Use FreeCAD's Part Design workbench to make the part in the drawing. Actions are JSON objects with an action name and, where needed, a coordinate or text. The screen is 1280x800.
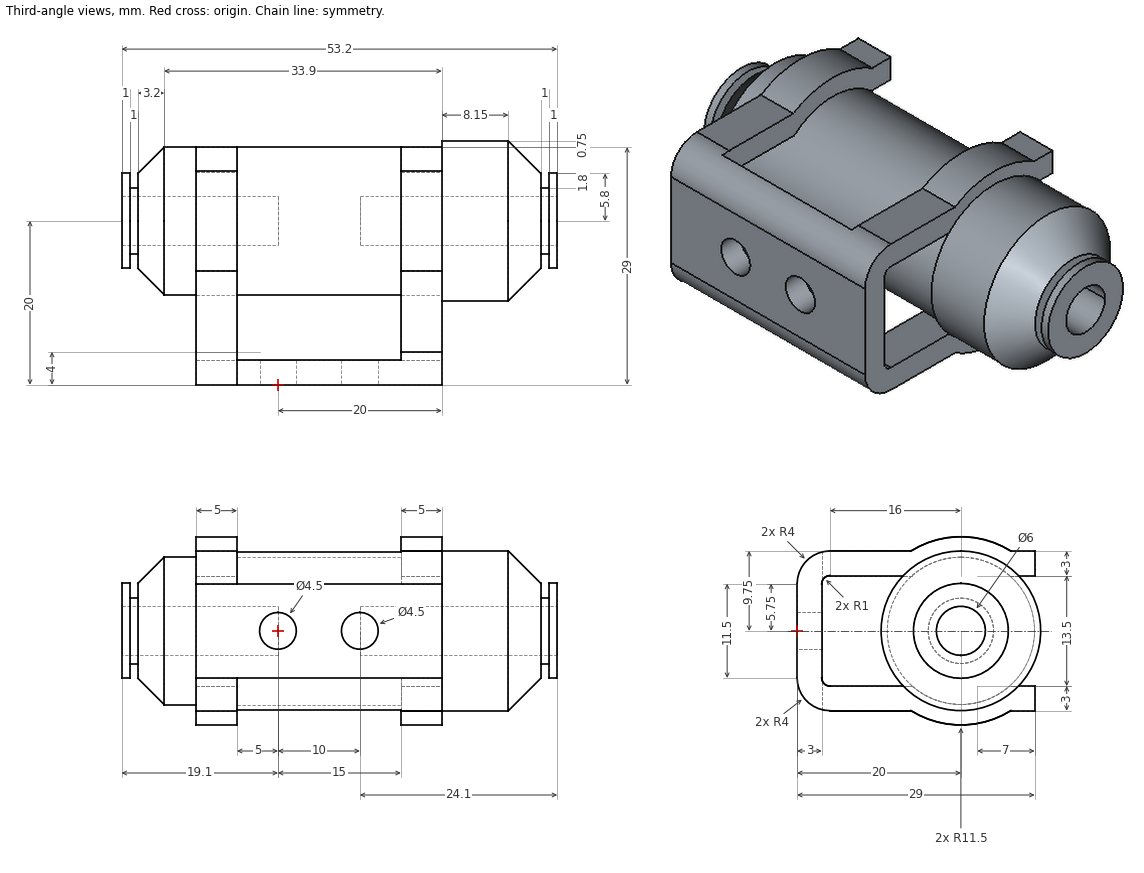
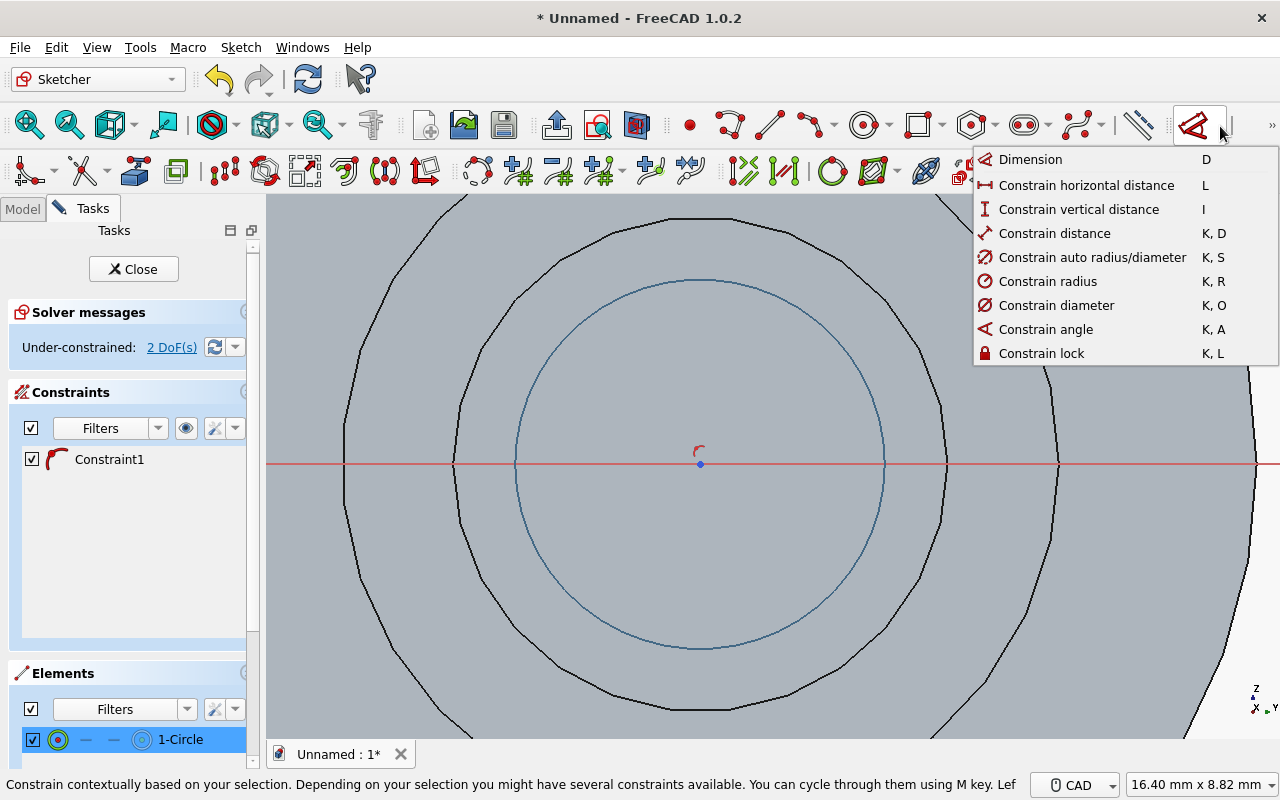
{"action": "left_click", "coordinate": [1126, 305]}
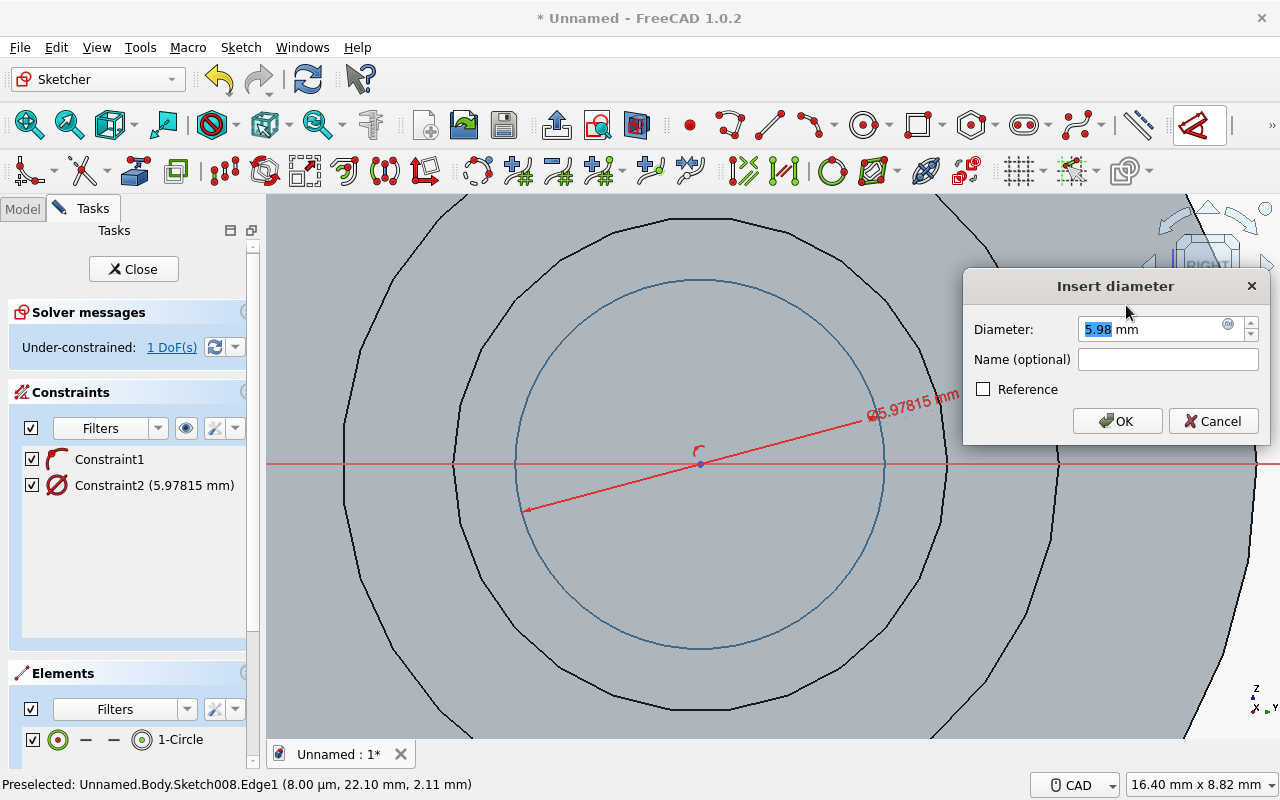
{"action": "type", "text": "6"}
{"action": "key", "text": "Return"}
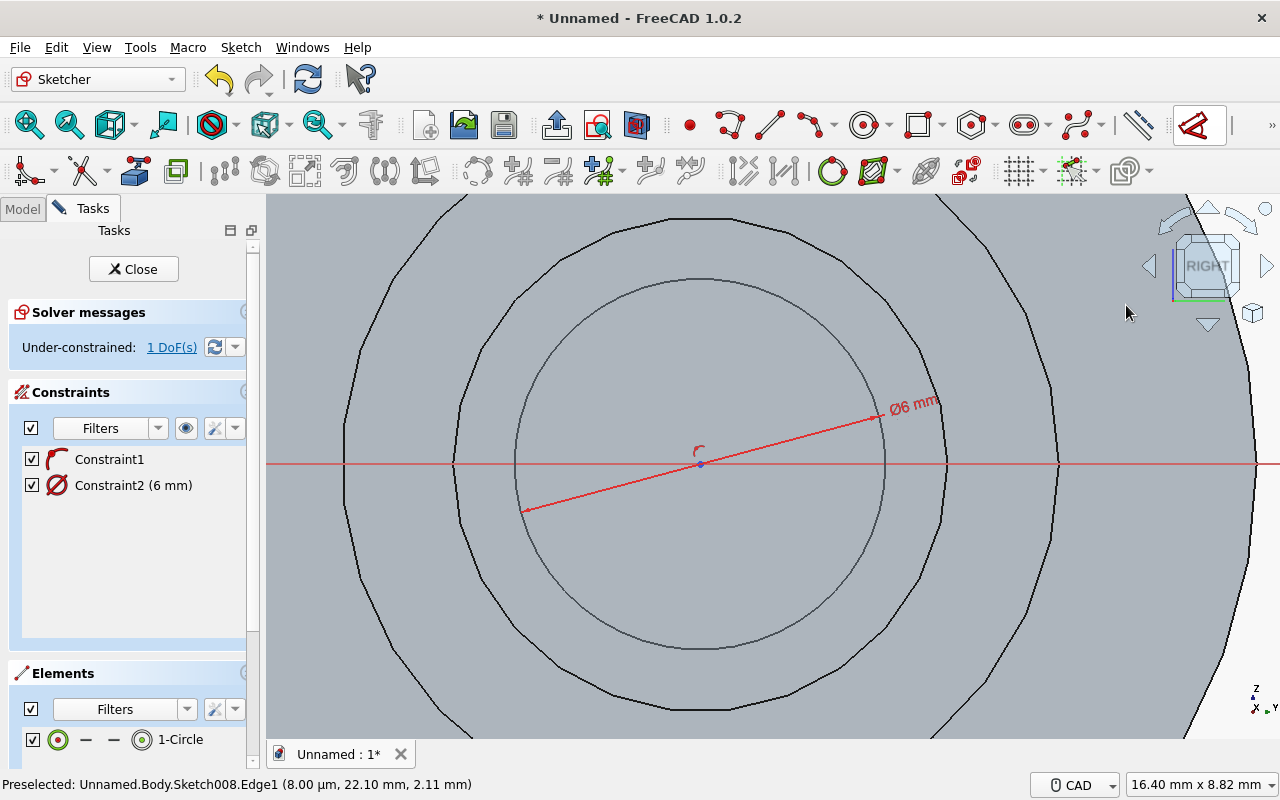
{"action": "left_click", "coordinate": [700, 464]}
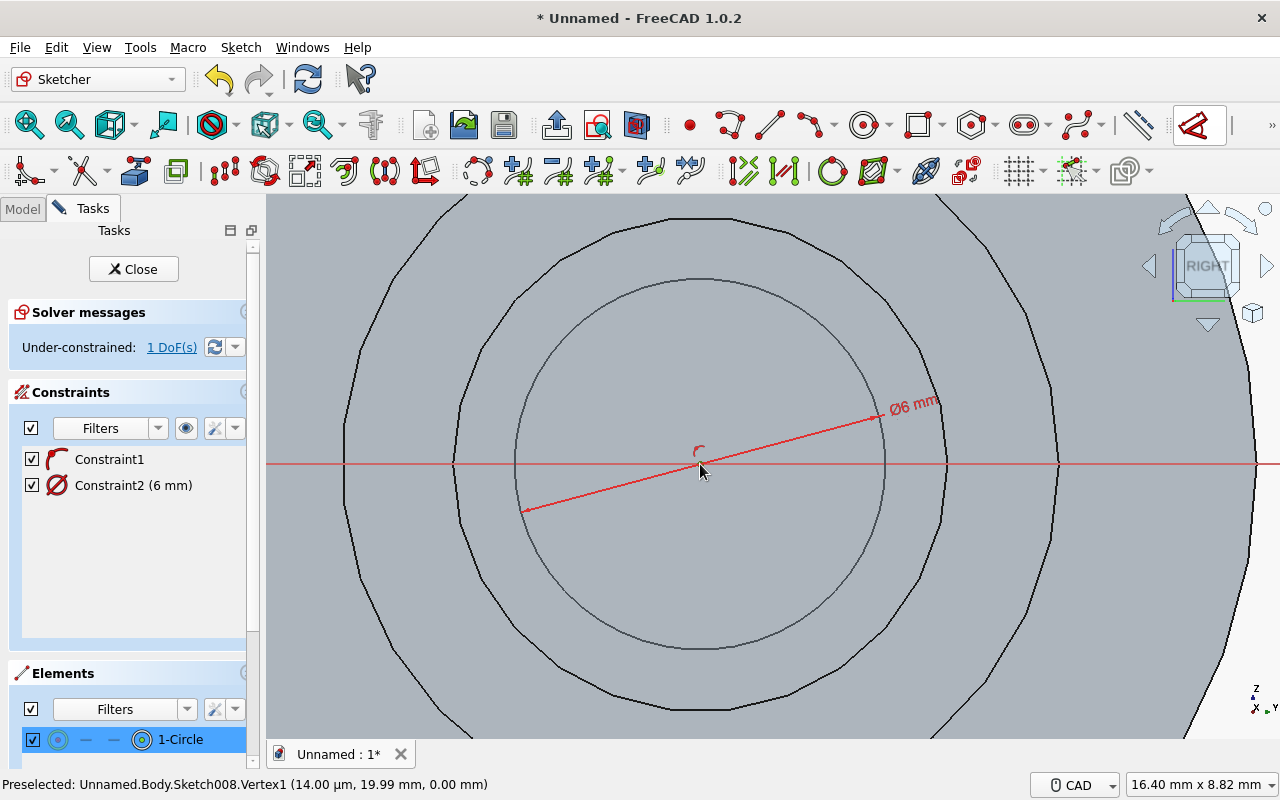
{"action": "left_click", "coordinate": [1220, 126]}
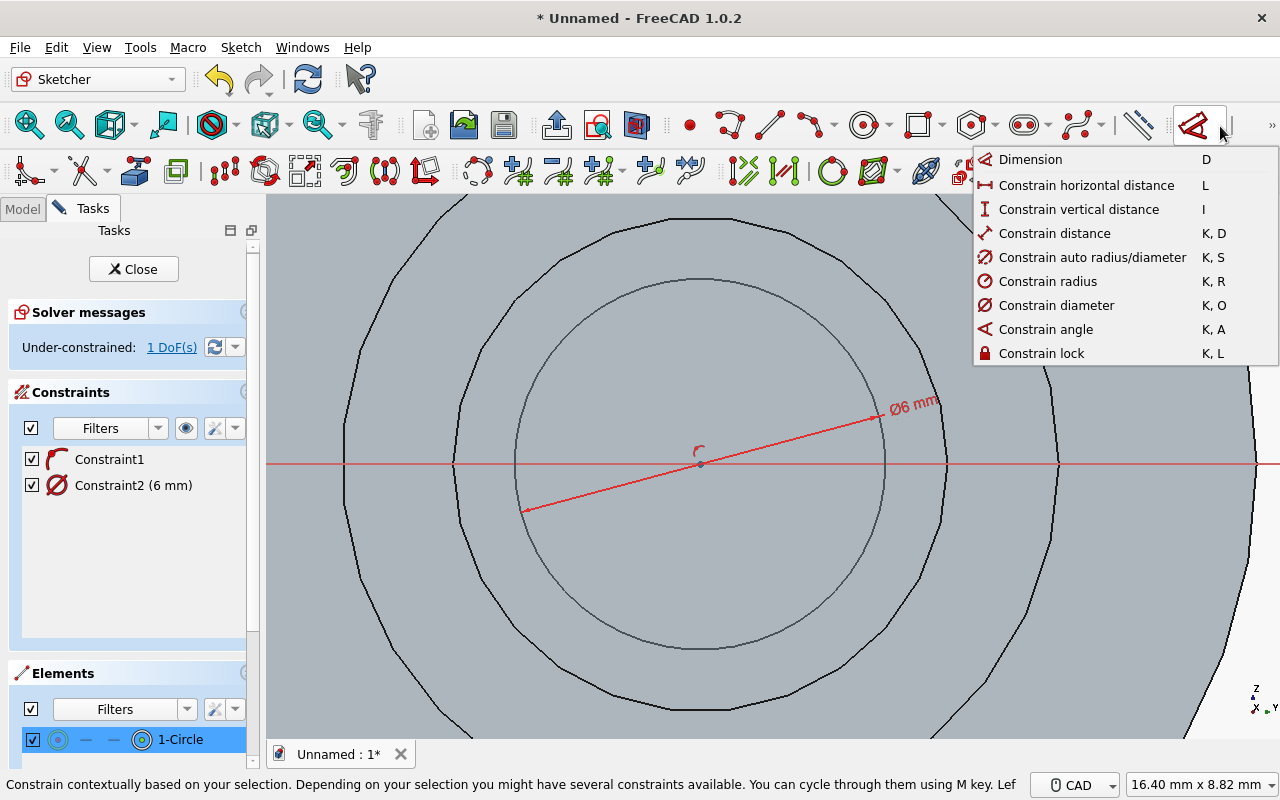
{"action": "left_click", "coordinate": [1126, 185]}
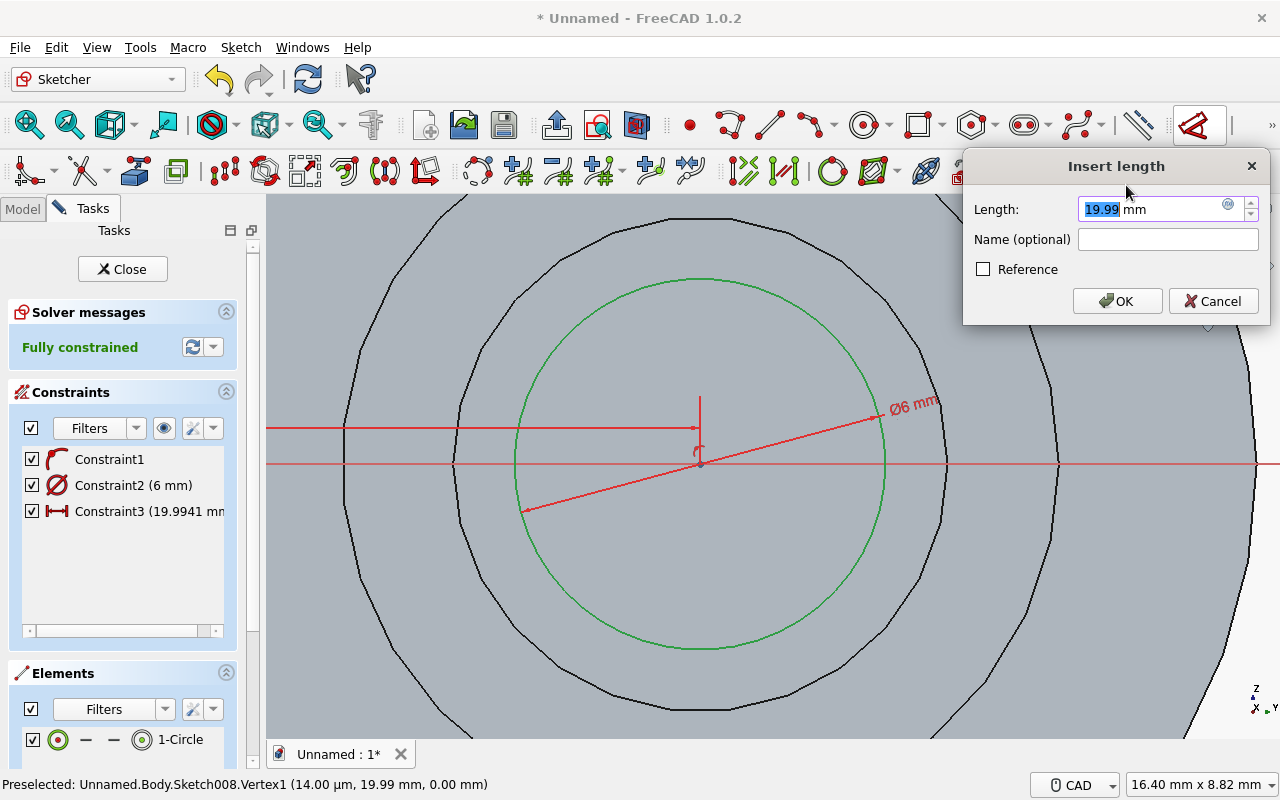
{"action": "type", "text": "20"}
{"action": "key", "text": "Return"}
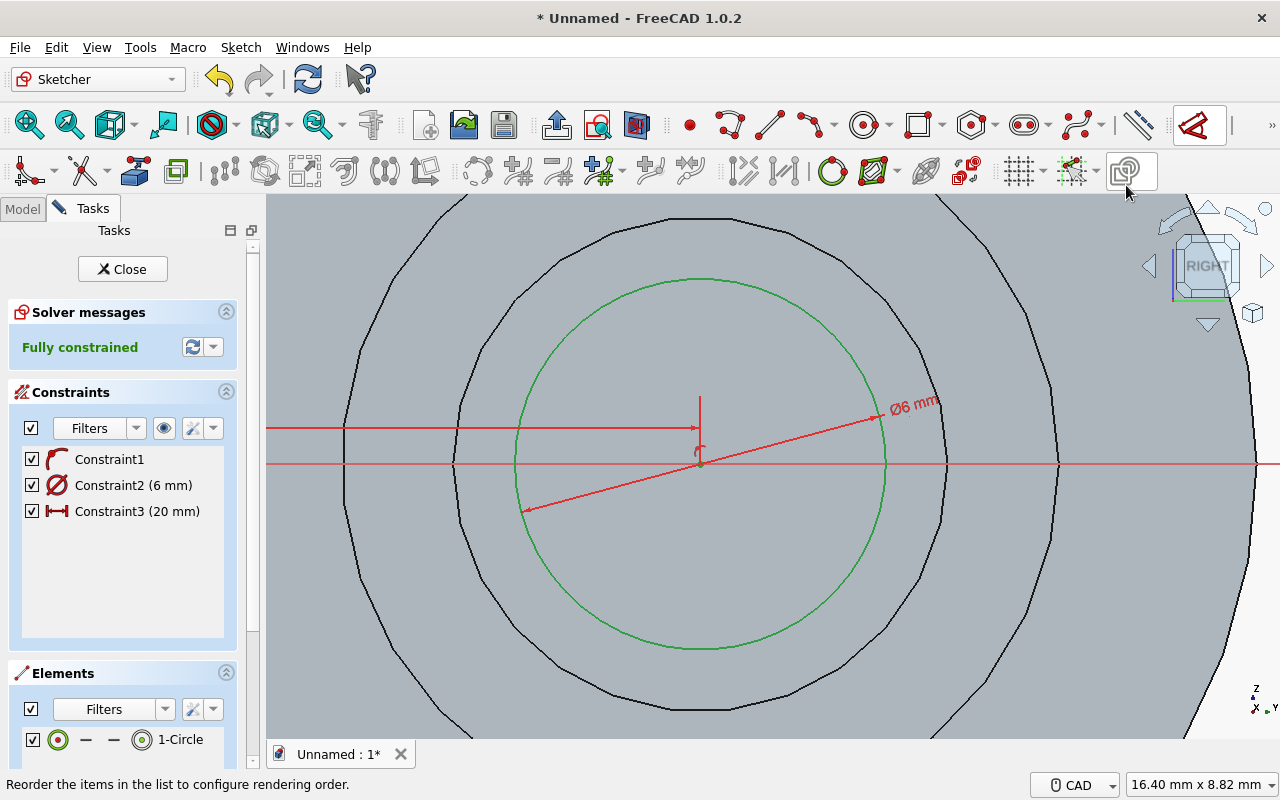
{"action": "left_click", "coordinate": [123, 269]}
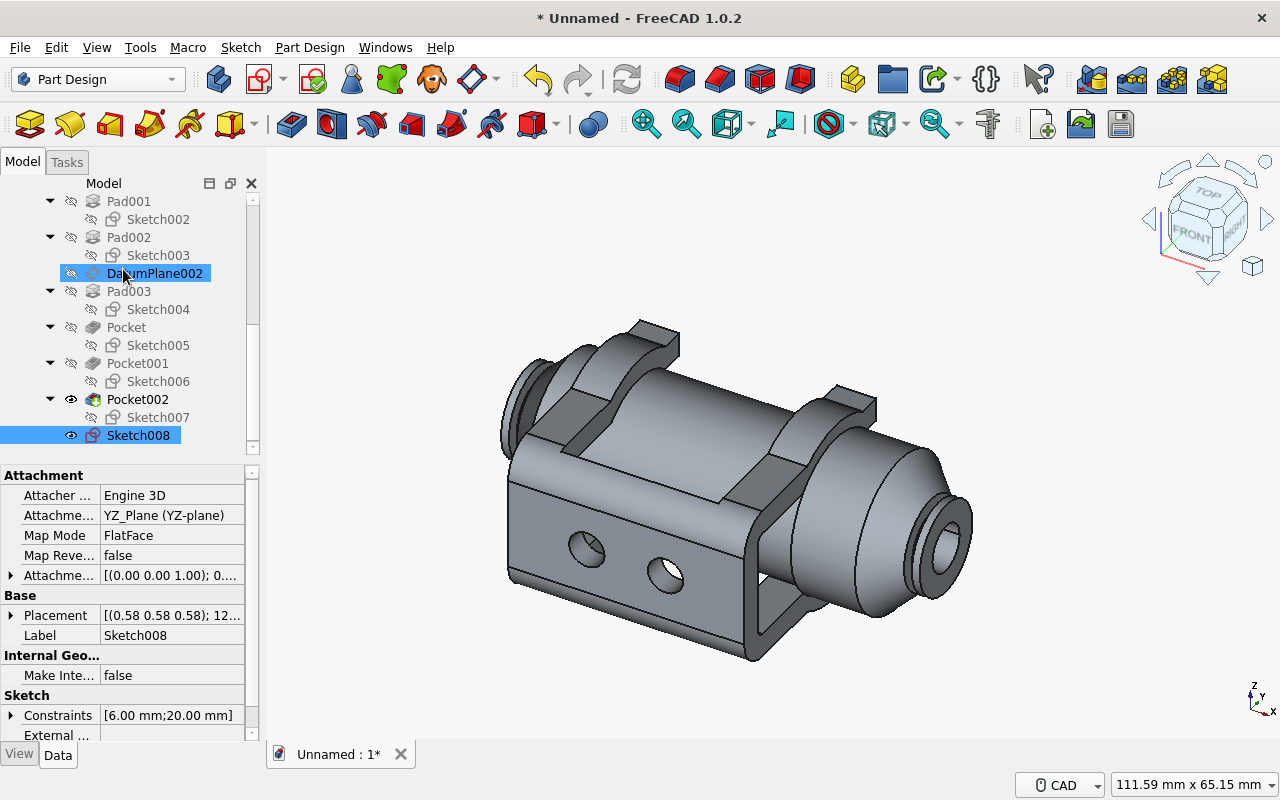
{"action": "left_click", "coordinate": [292, 124]}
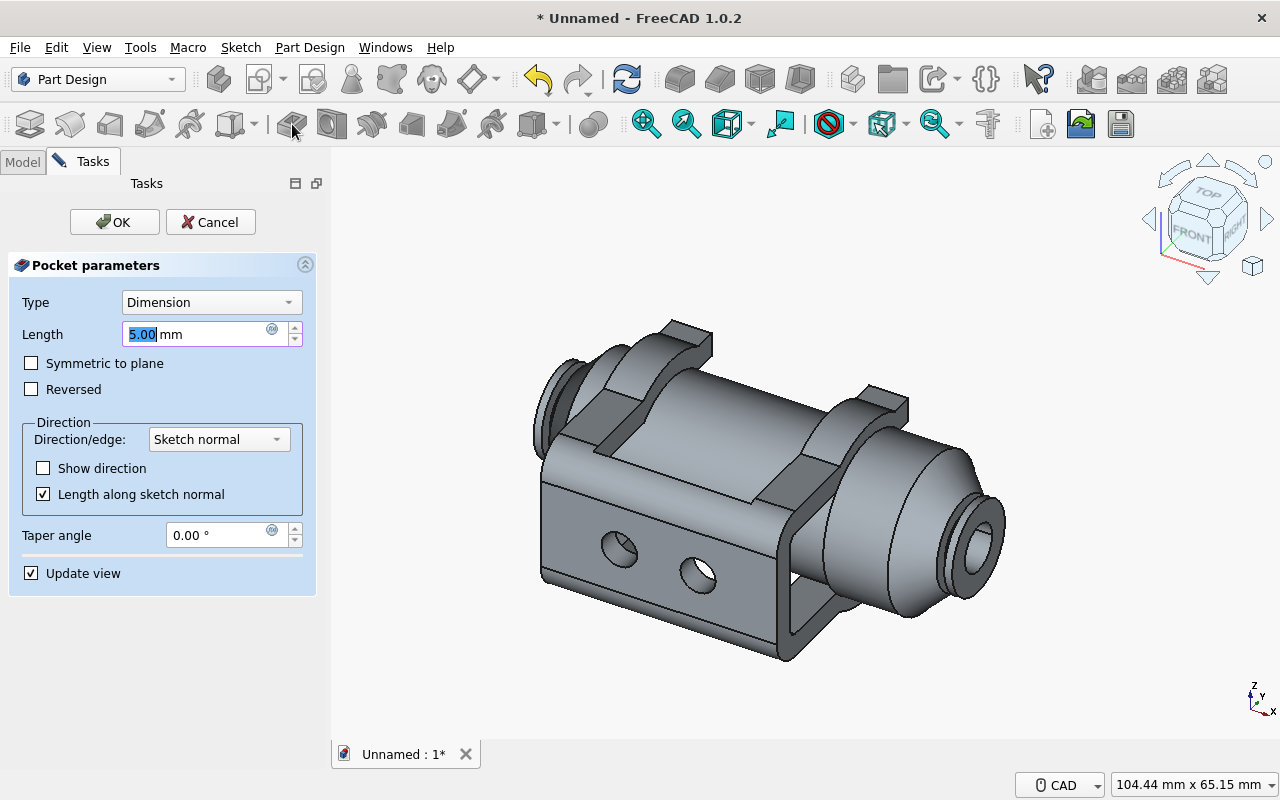
{"action": "type", "text": "19.1"}
{"action": "key", "text": "Tab"}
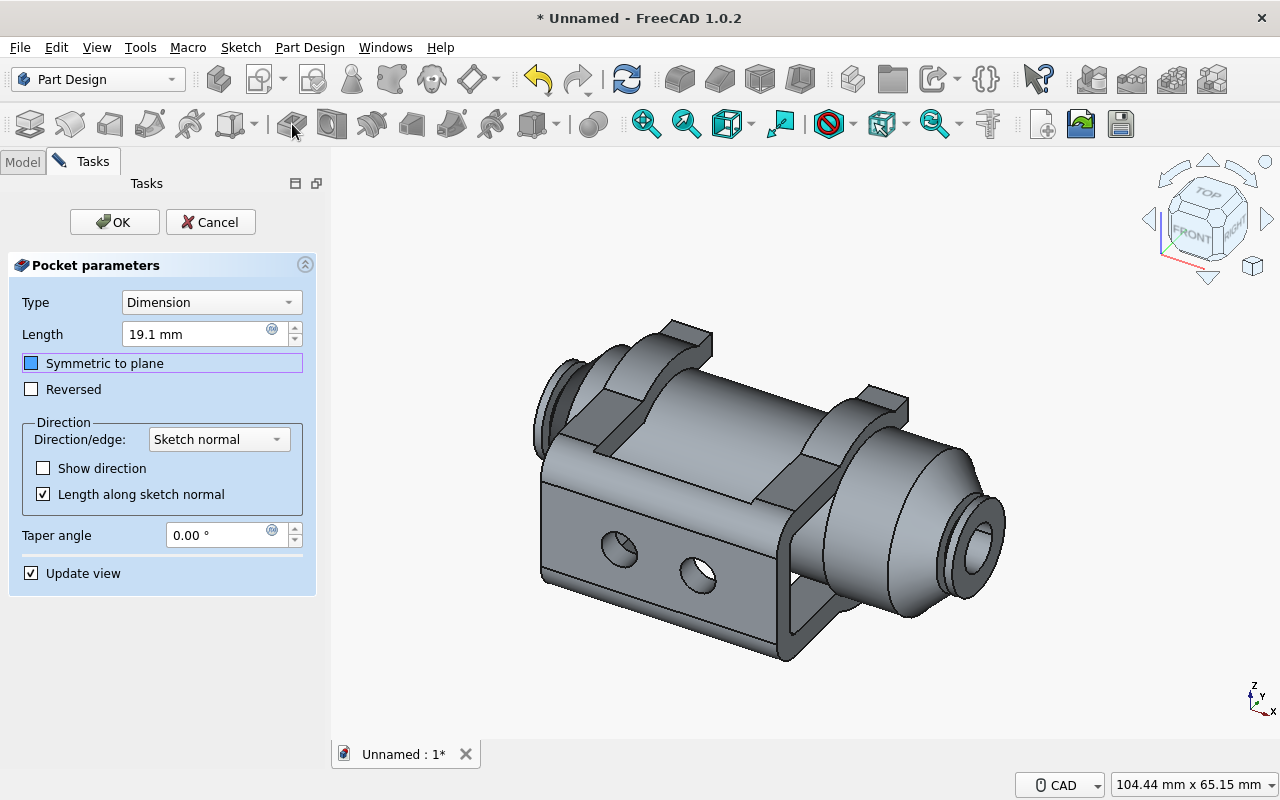
{"action": "left_click", "coordinate": [115, 222]}